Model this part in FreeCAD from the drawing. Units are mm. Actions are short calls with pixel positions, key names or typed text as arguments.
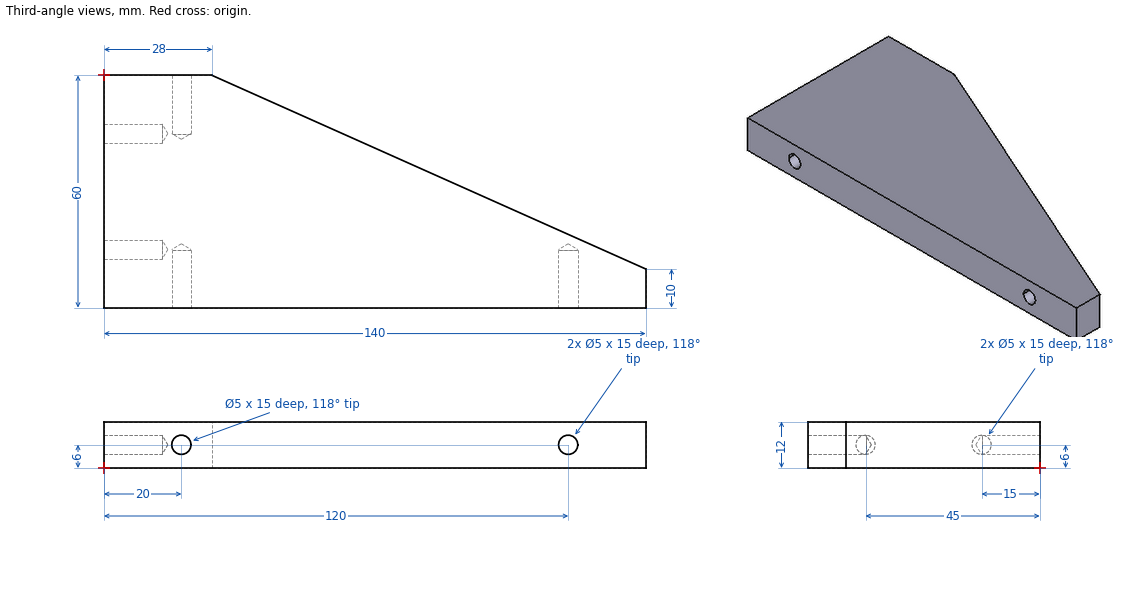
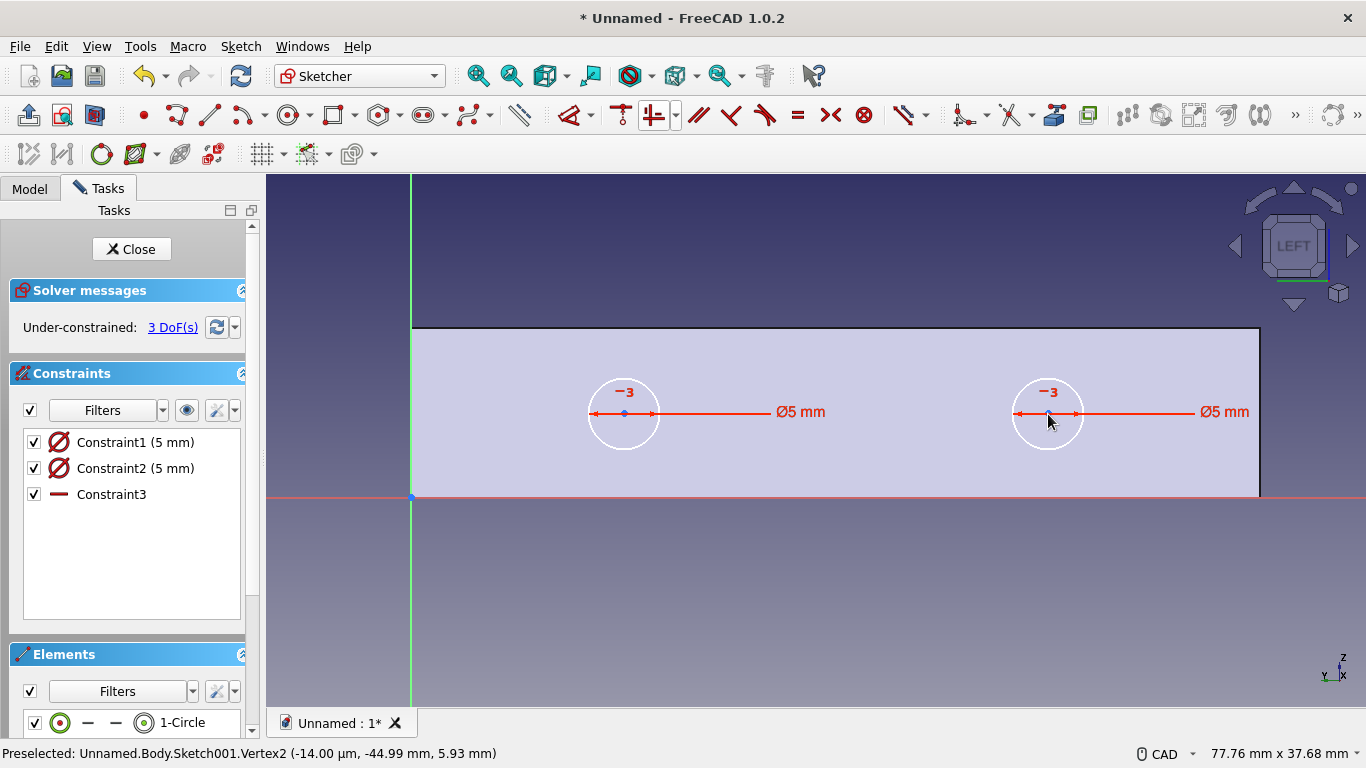
key(d)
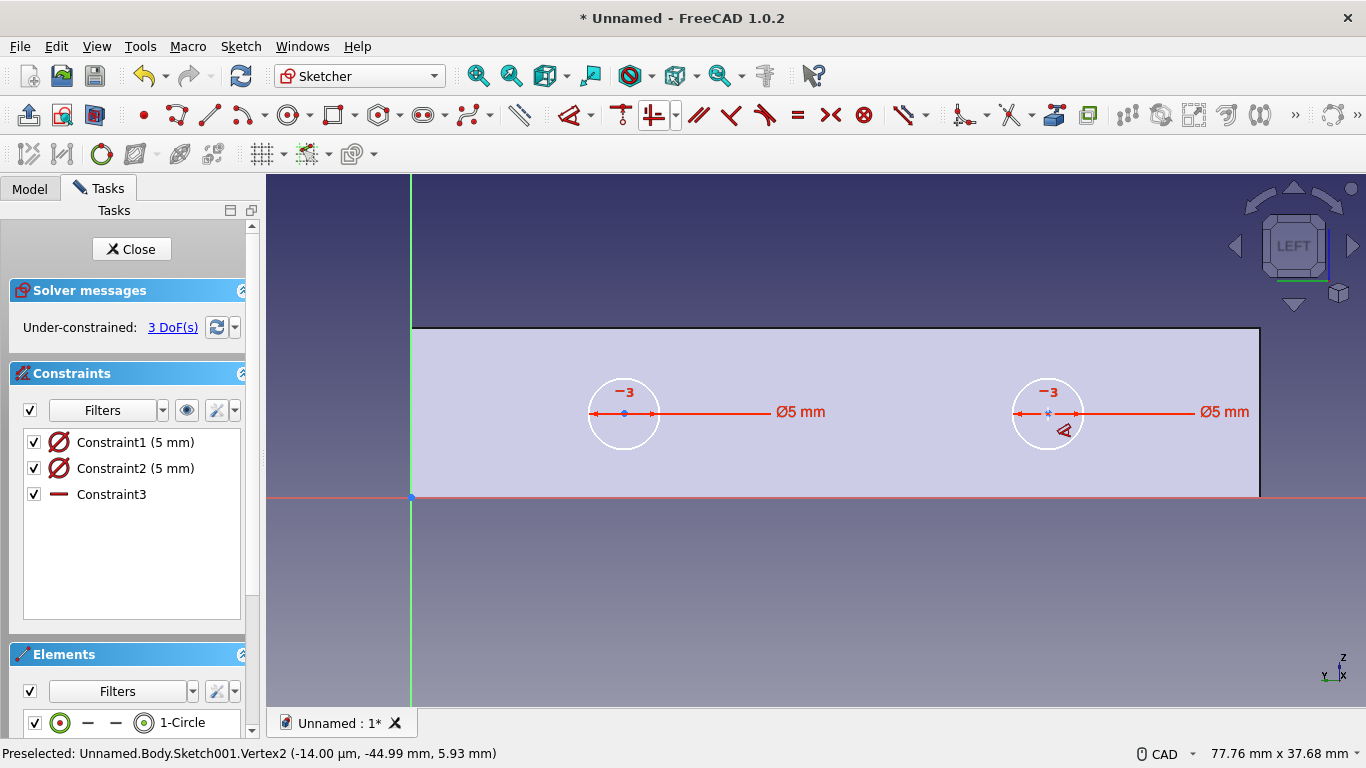
click(624, 414)
click(377, 456)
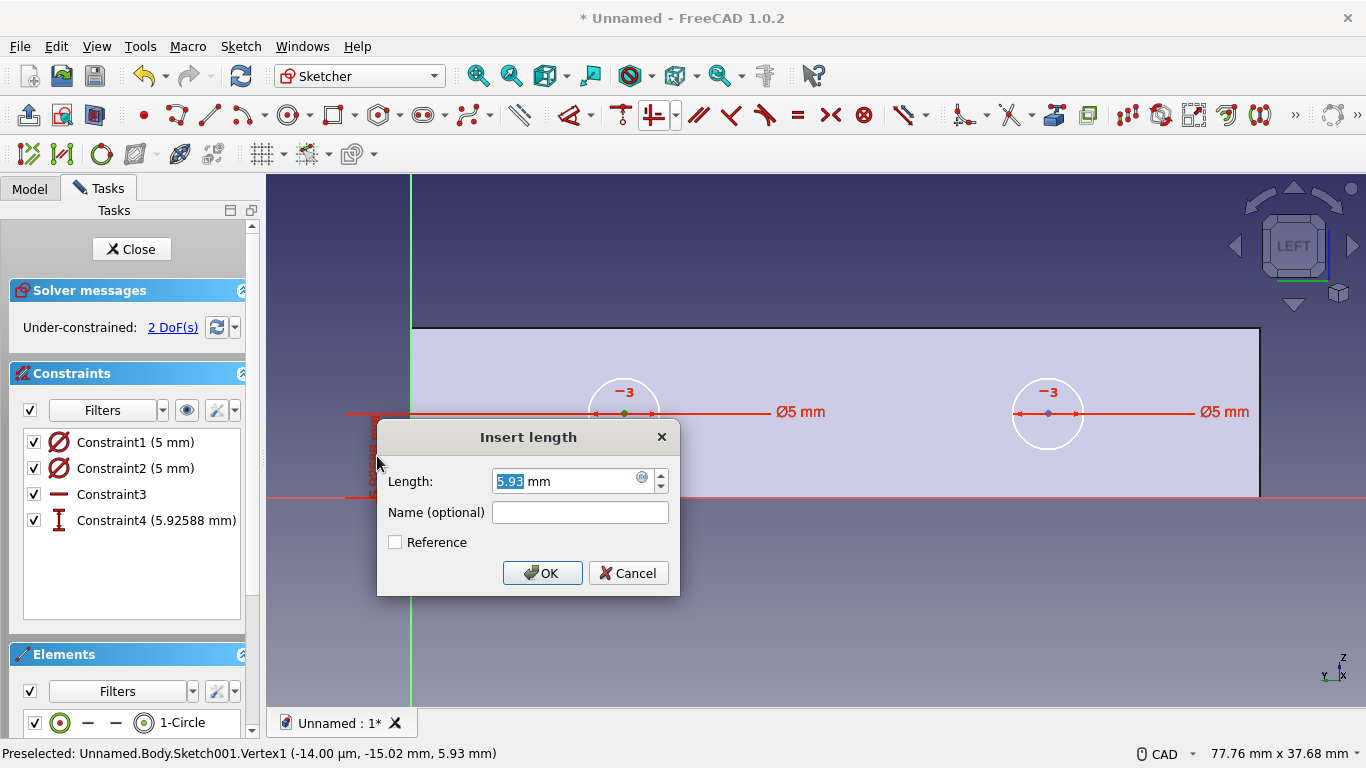
text(6)
key(Return)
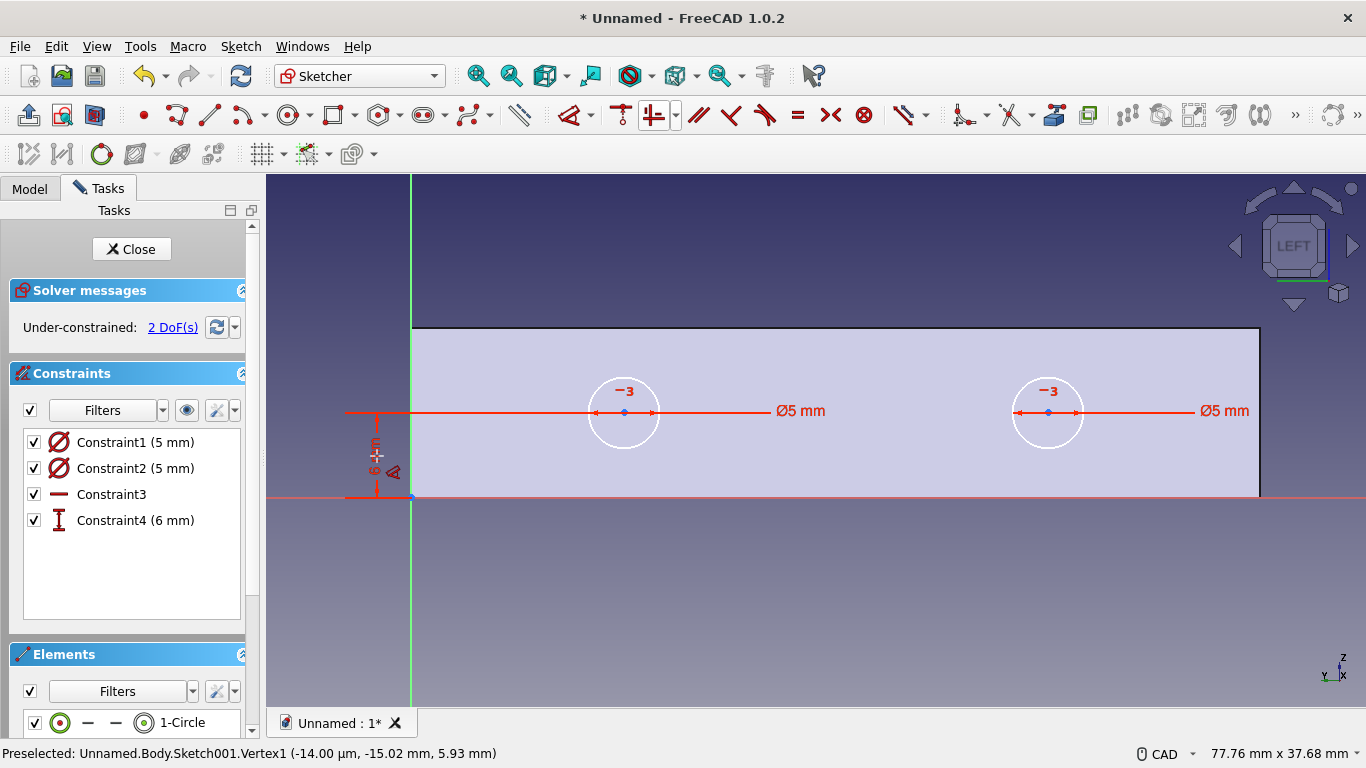
click(624, 413)
click(518, 532)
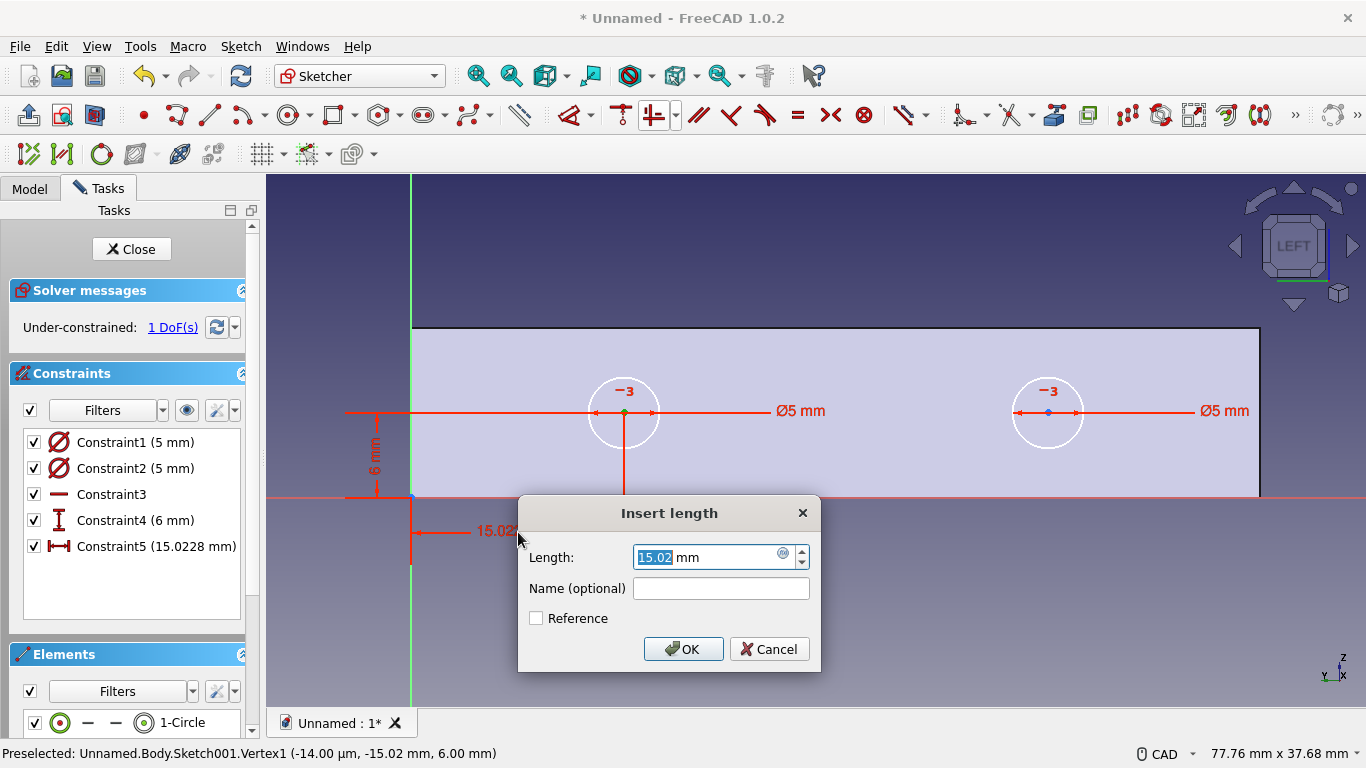
text(15)
key(Return)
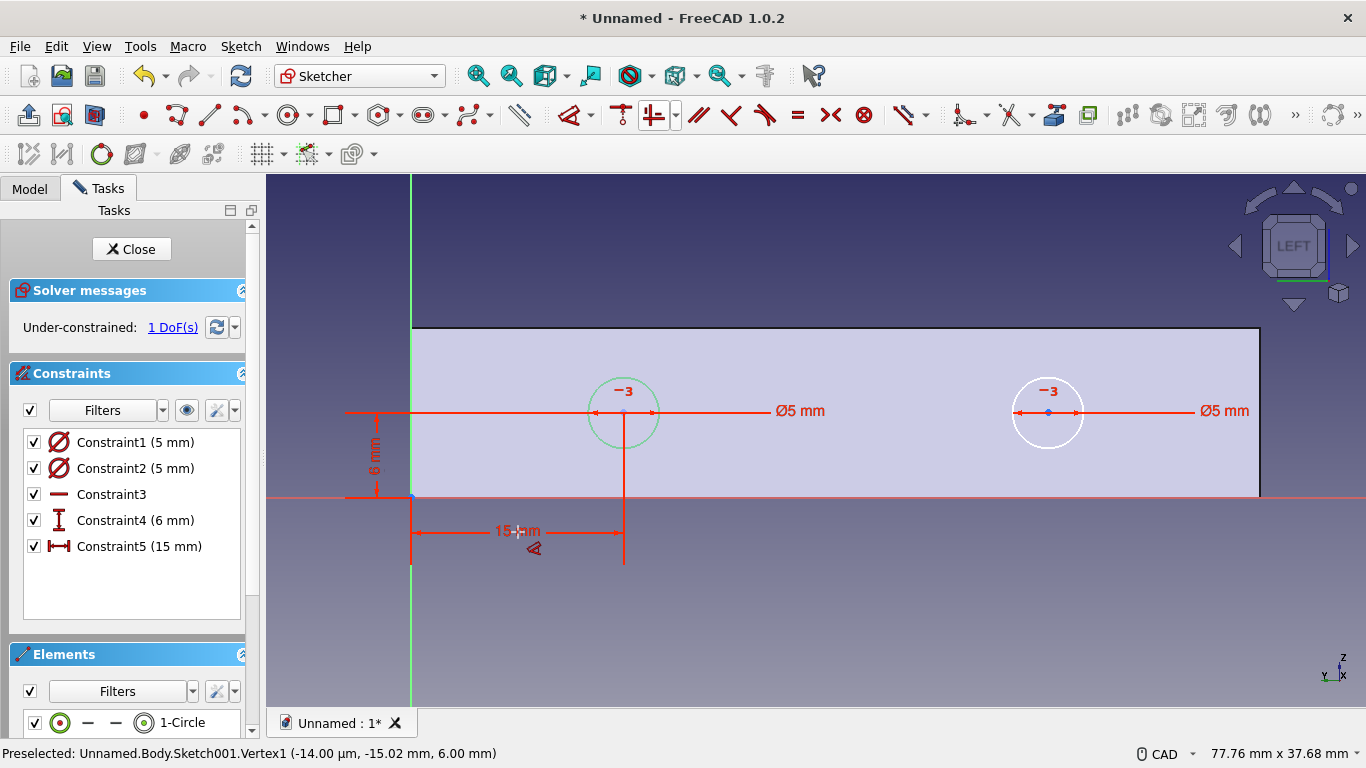
click(1048, 413)
click(730, 532)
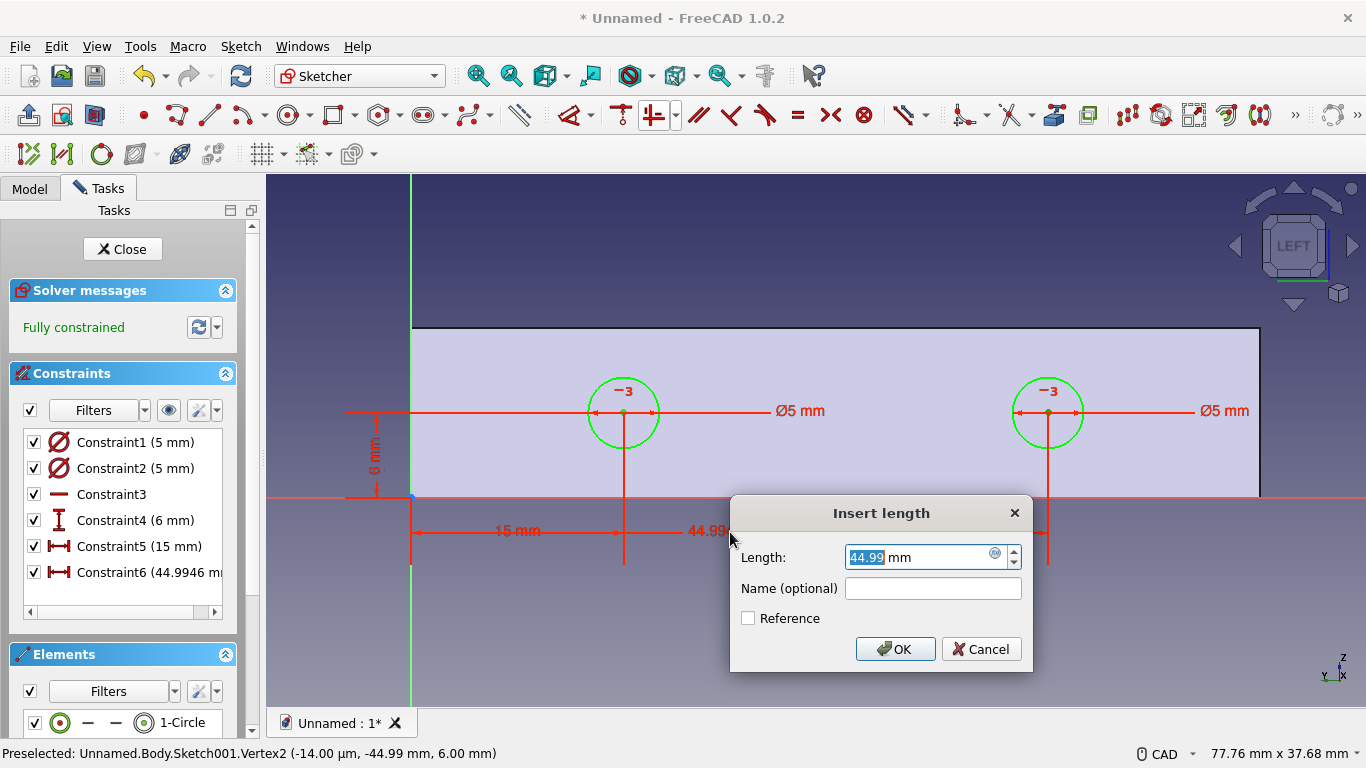
text(45)
key(Return)
key(Escape)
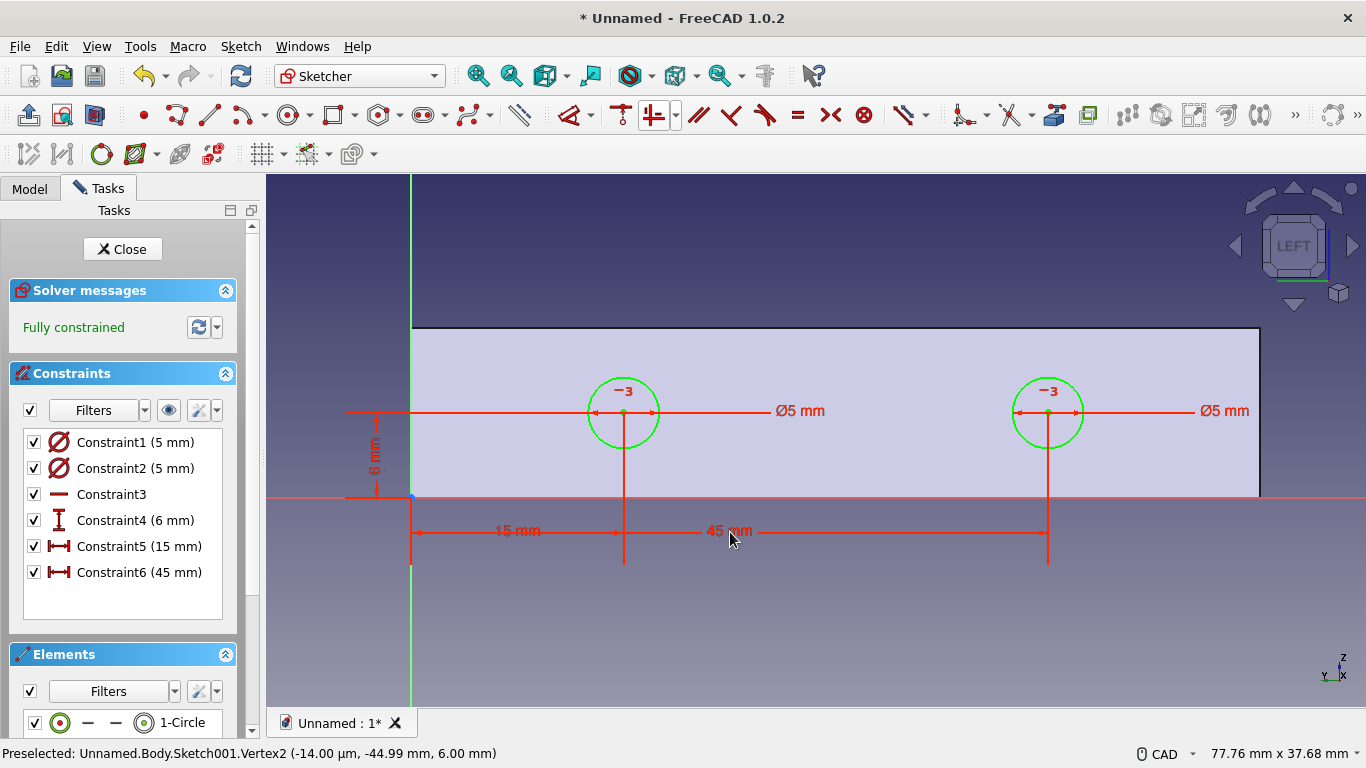
click(123, 249)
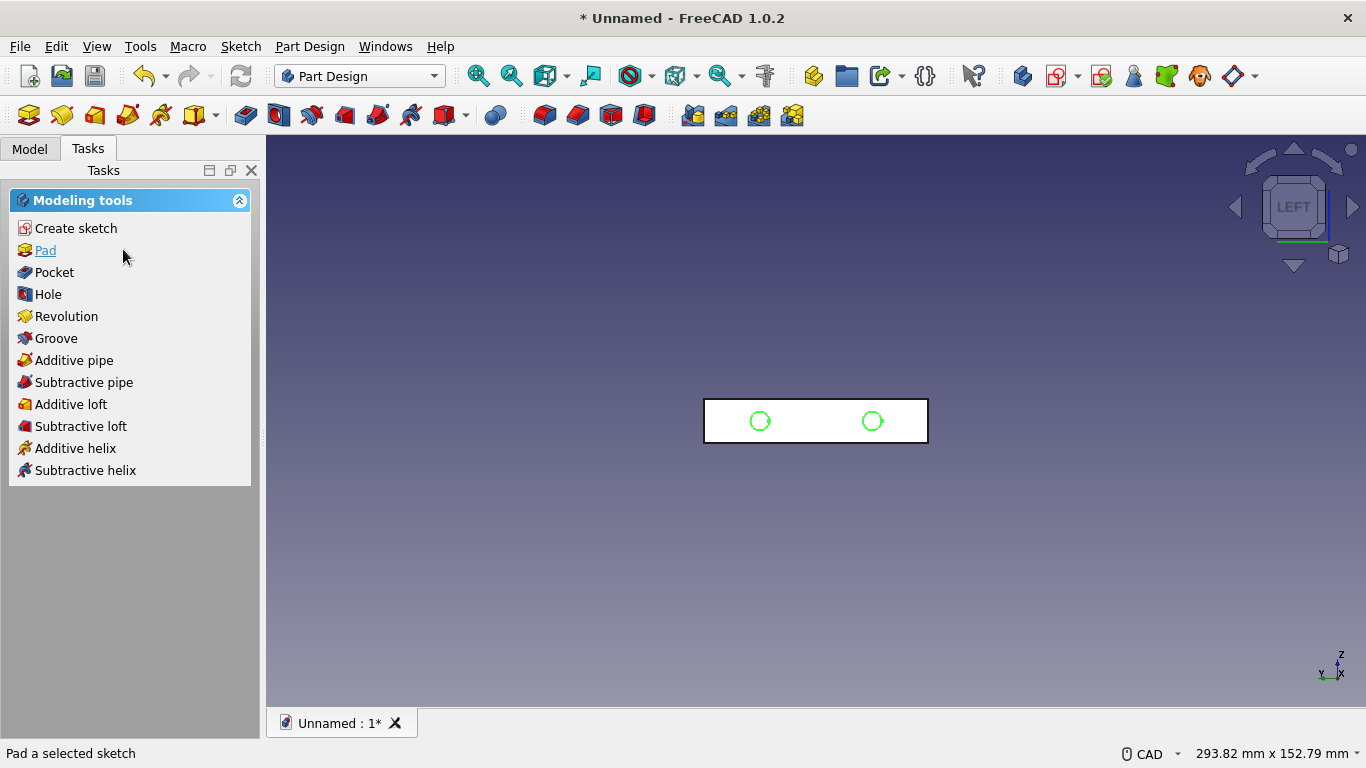
click(279, 116)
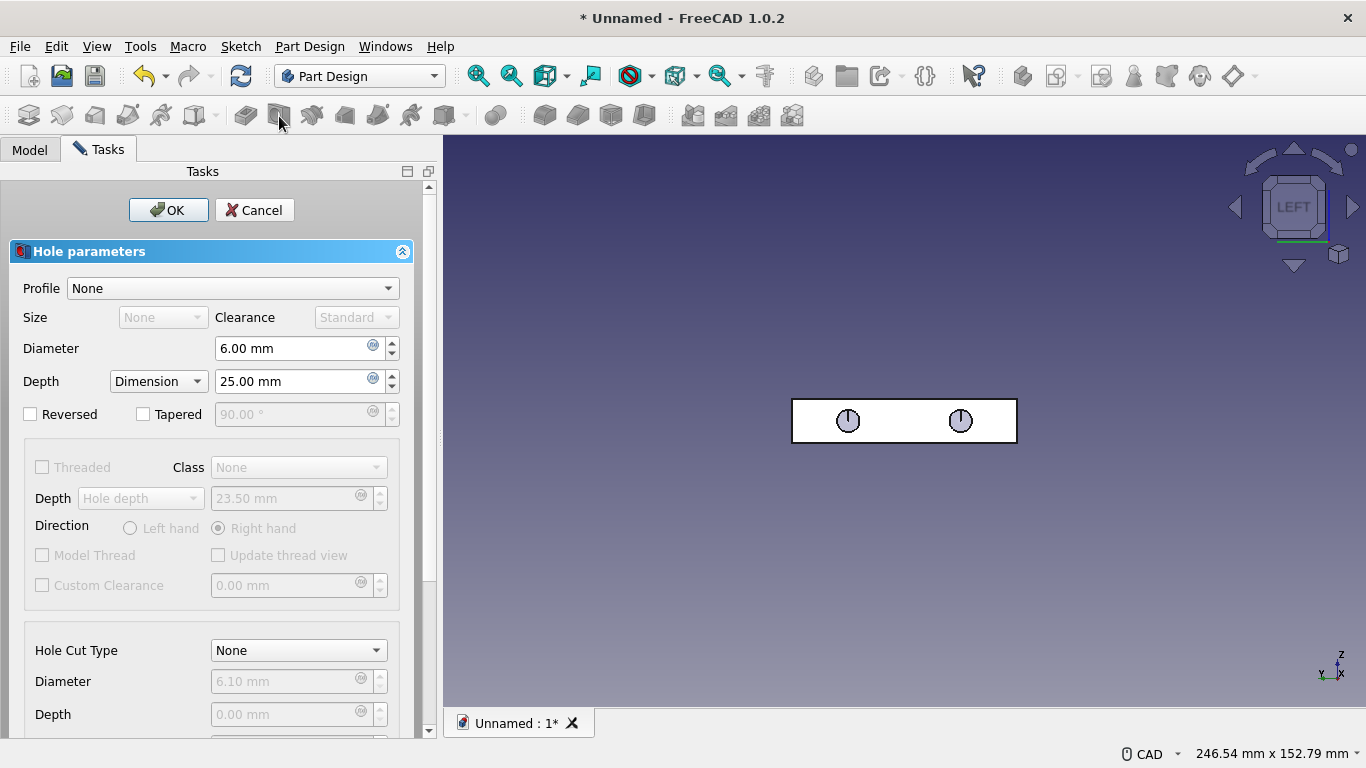
triple_click(300, 348)